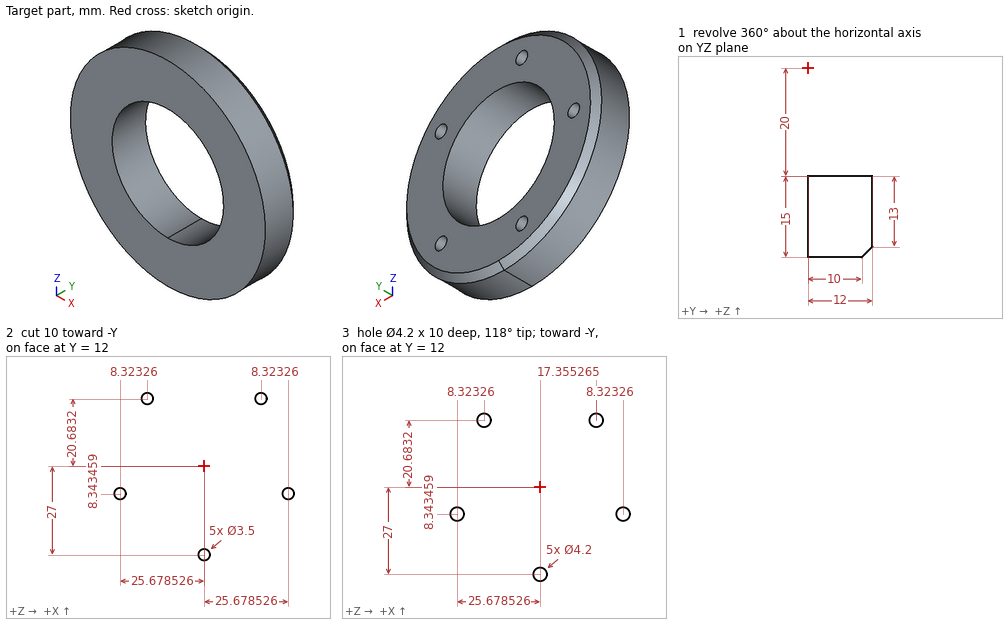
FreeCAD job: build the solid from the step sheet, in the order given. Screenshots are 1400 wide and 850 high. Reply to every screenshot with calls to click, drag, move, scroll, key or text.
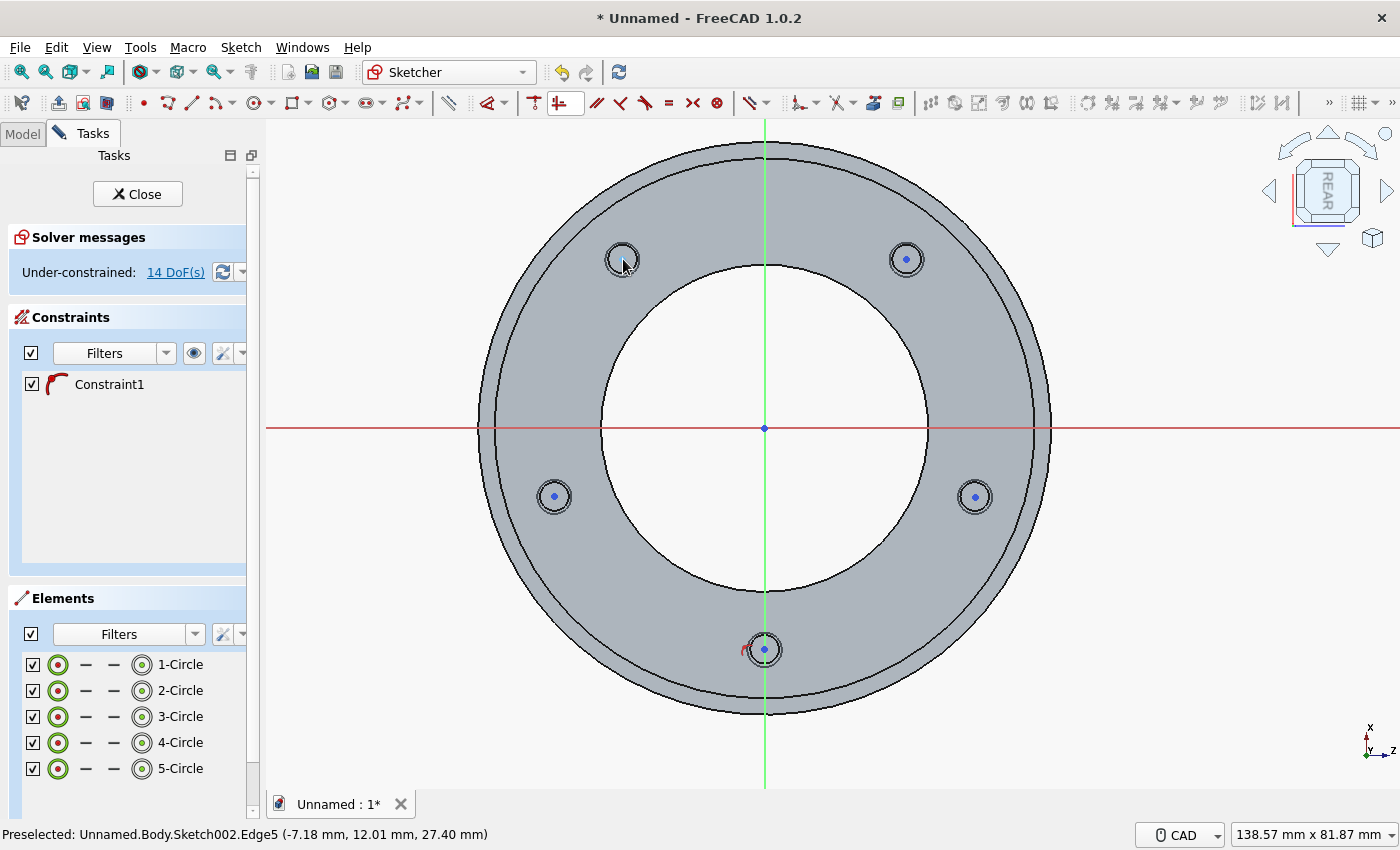
click(777, 638)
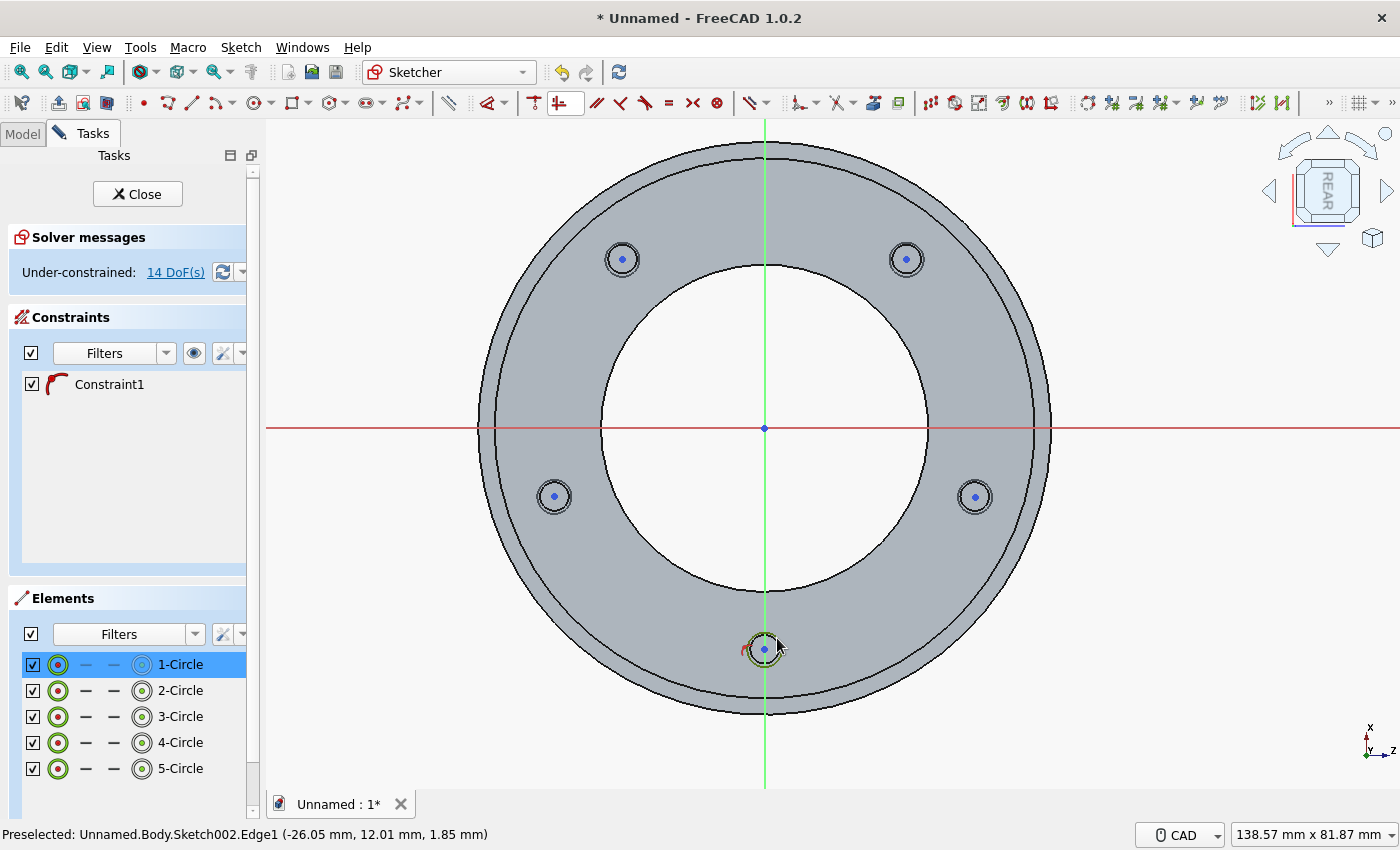
click(566, 485)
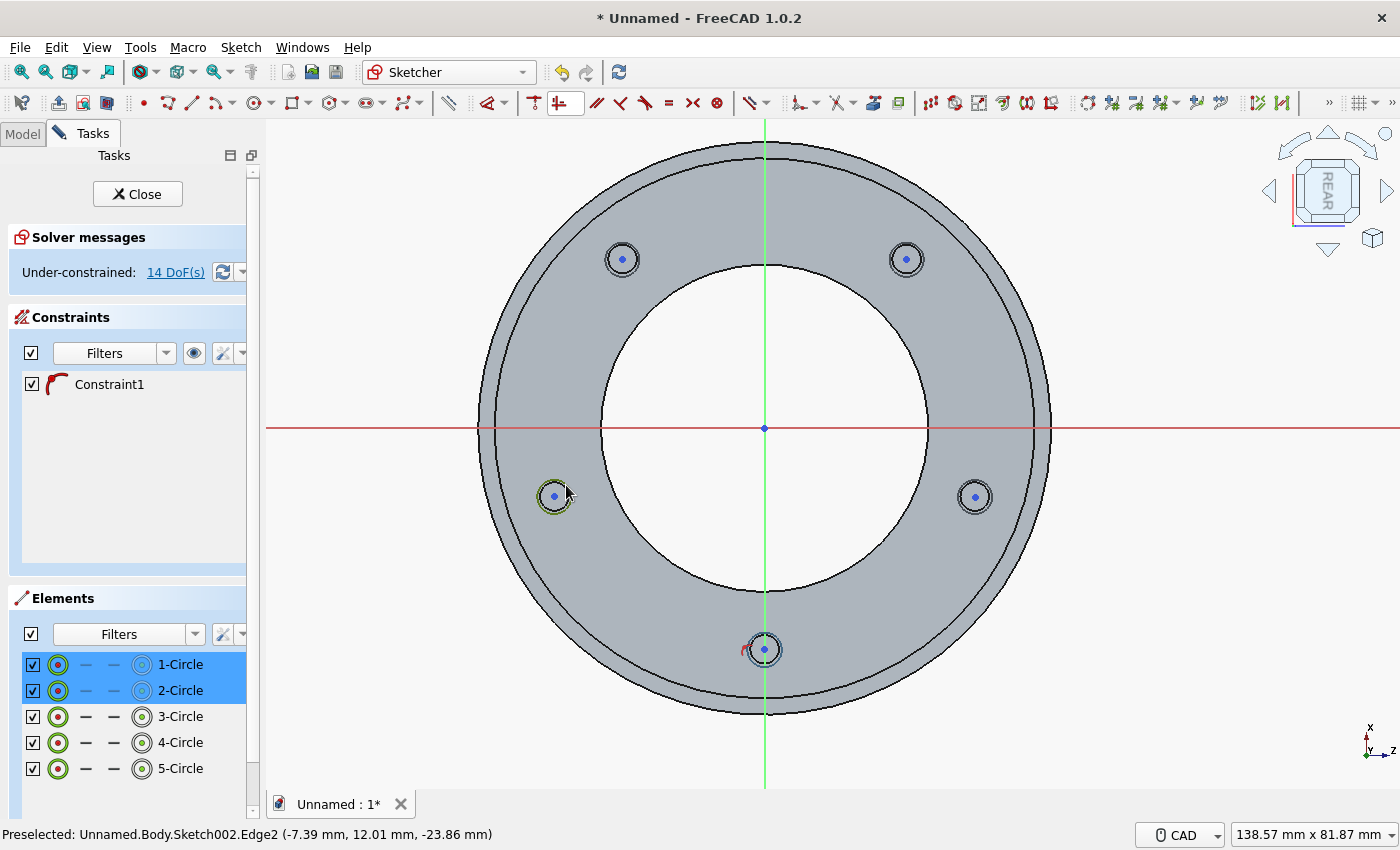
click(634, 248)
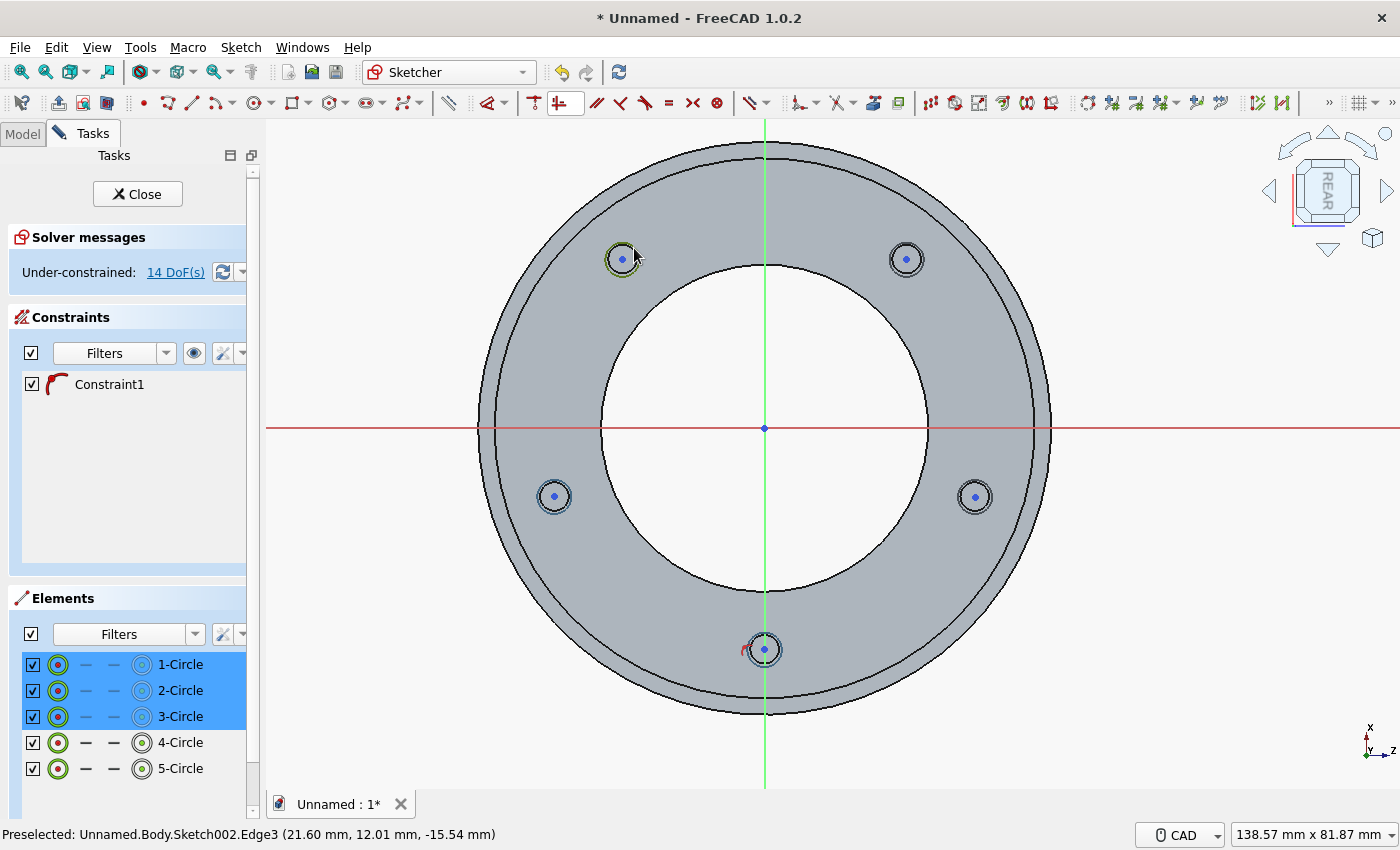
click(919, 248)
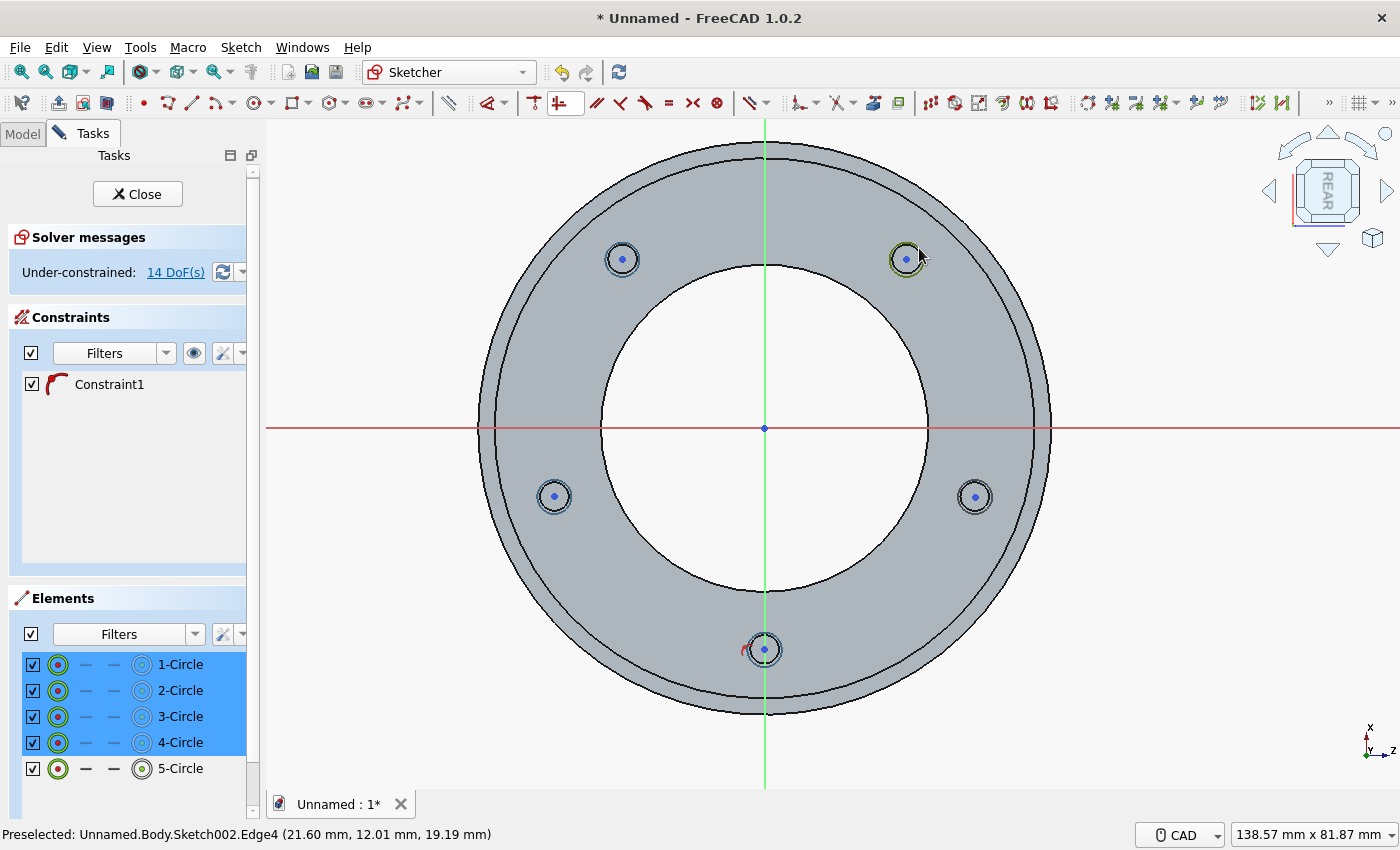
click(987, 485)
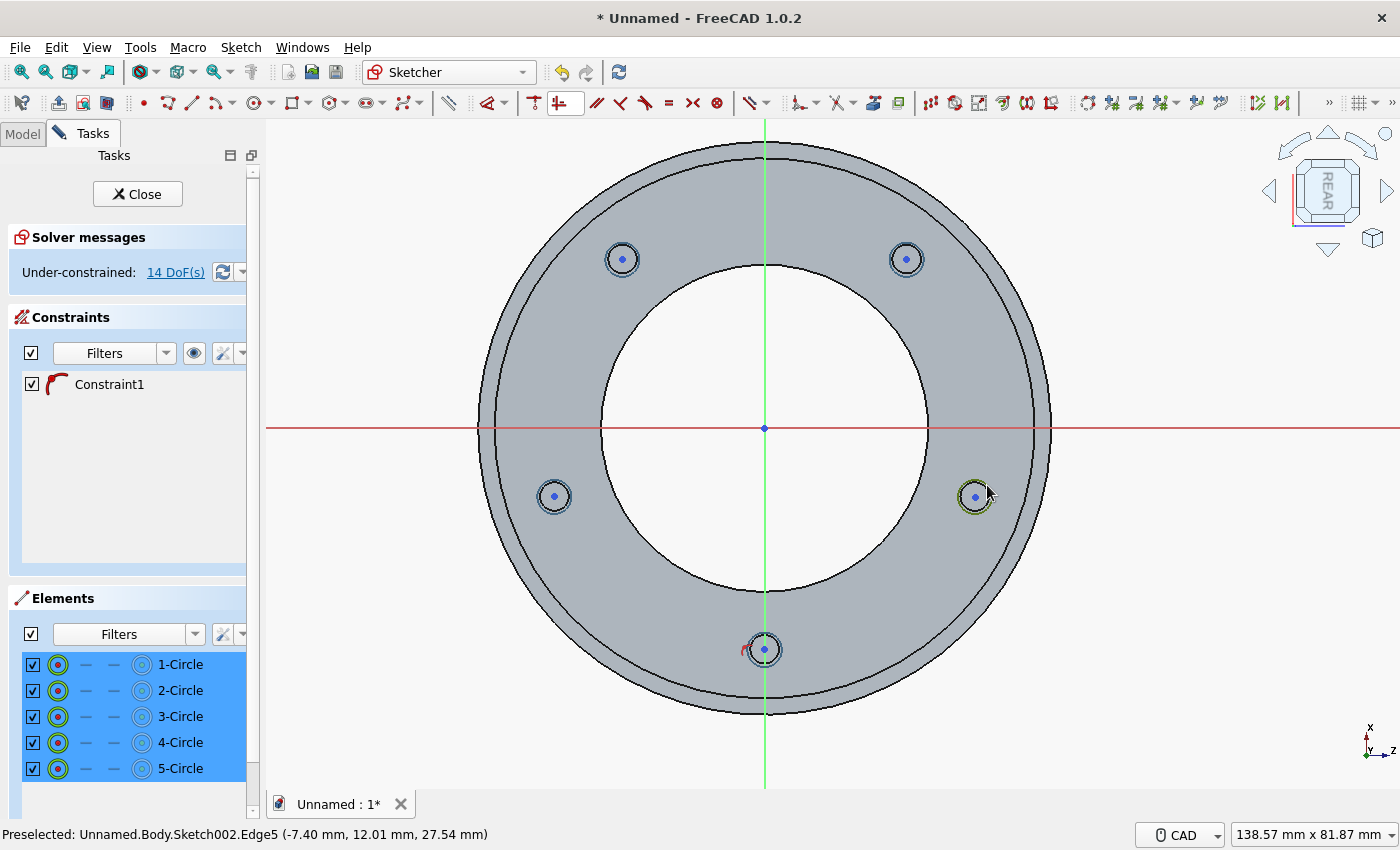
key(e)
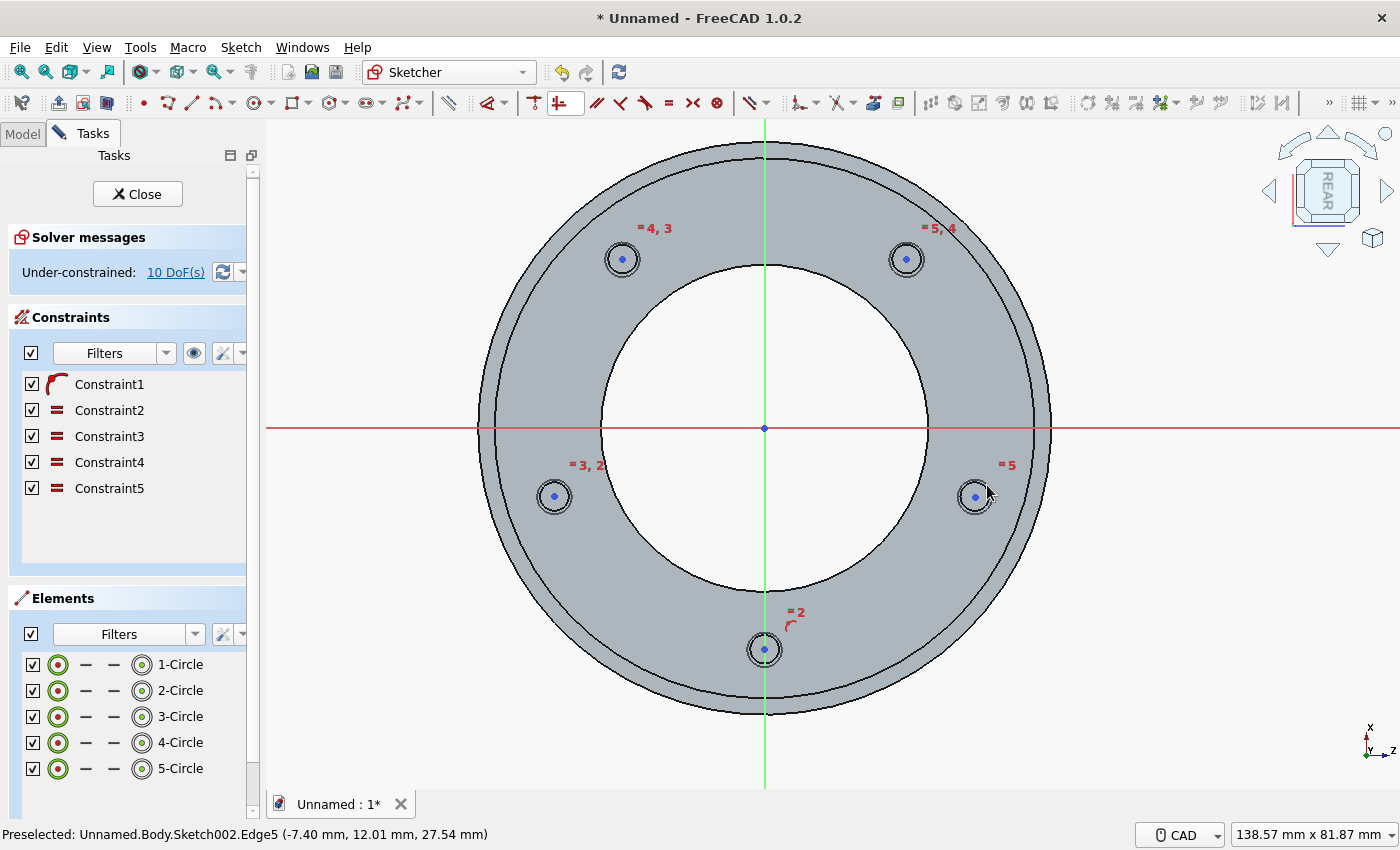
click(622, 260)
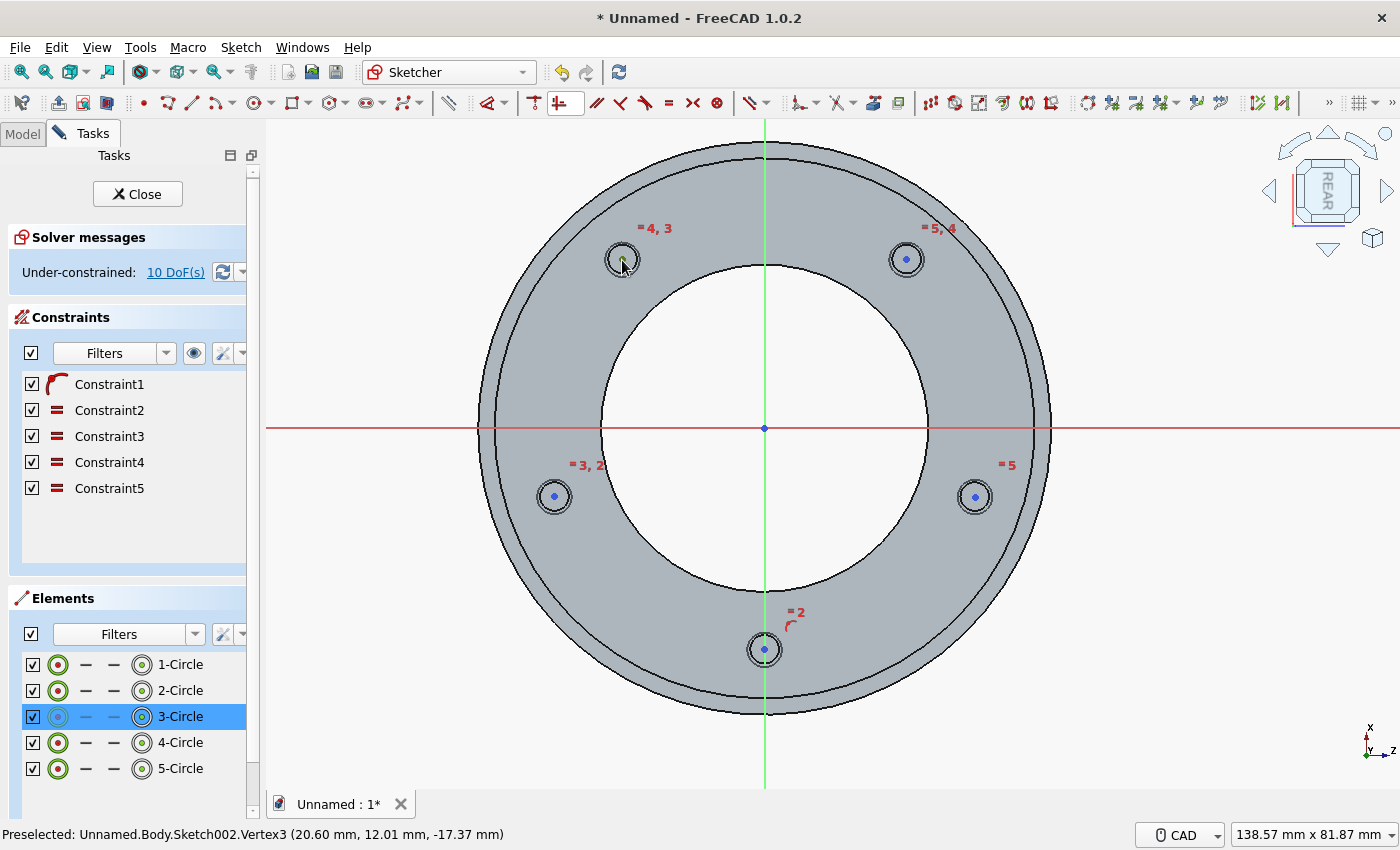
click(907, 260)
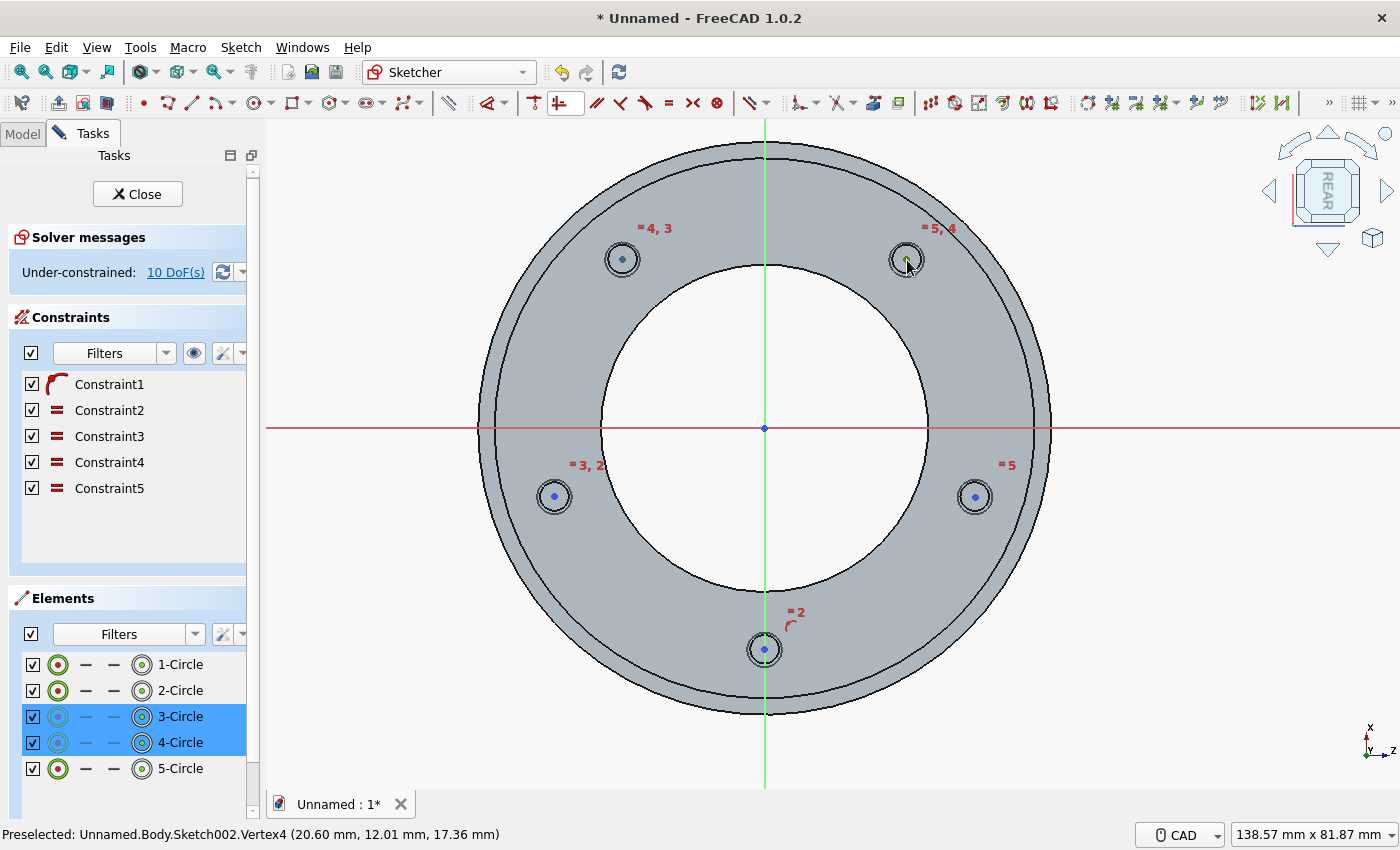
click(578, 104)